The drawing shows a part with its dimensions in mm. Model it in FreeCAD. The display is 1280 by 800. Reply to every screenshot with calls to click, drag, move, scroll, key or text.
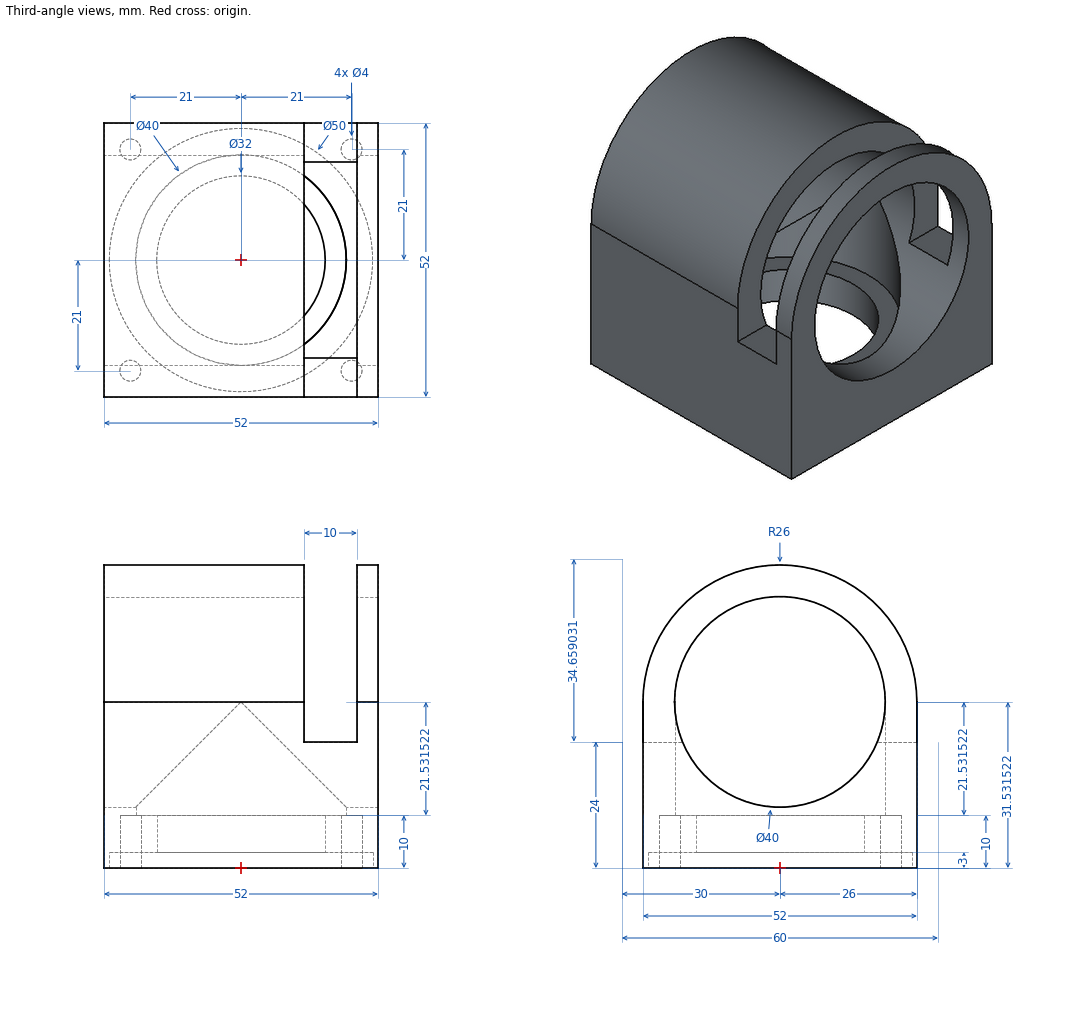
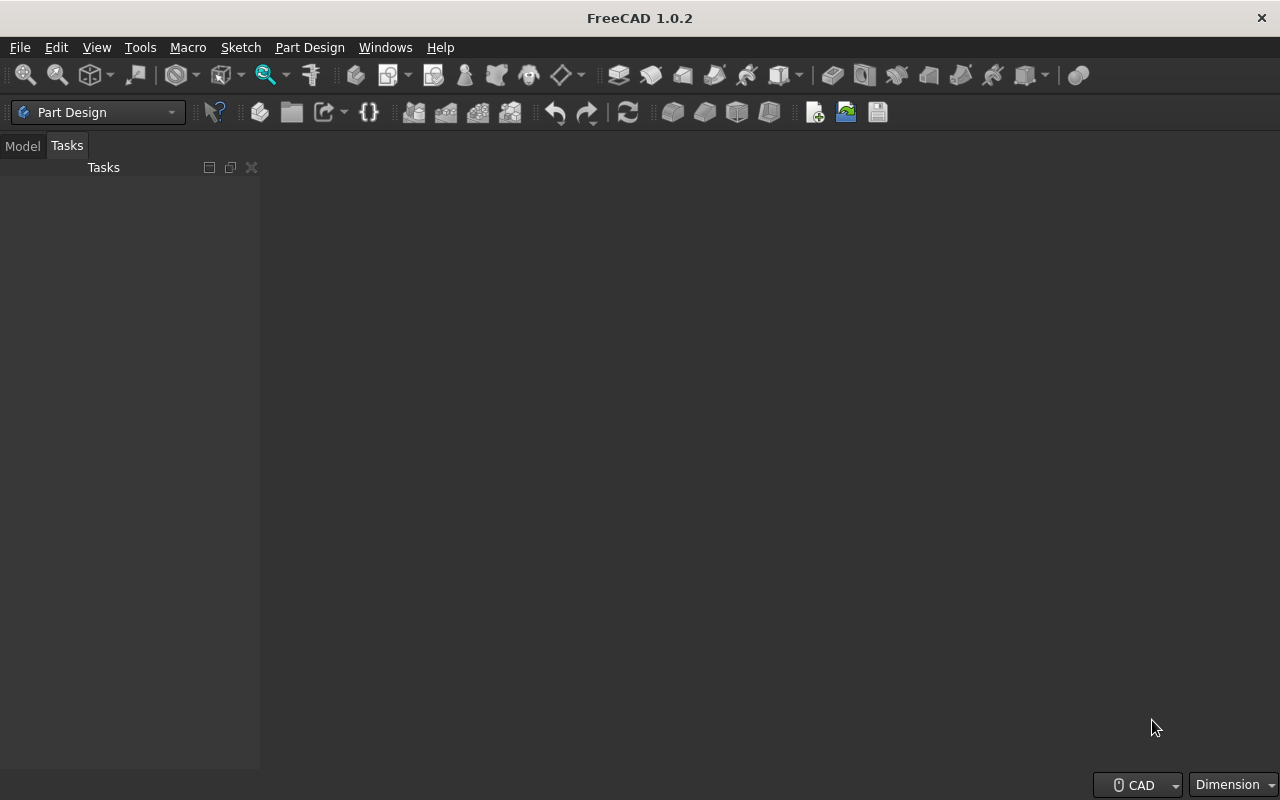
click(814, 112)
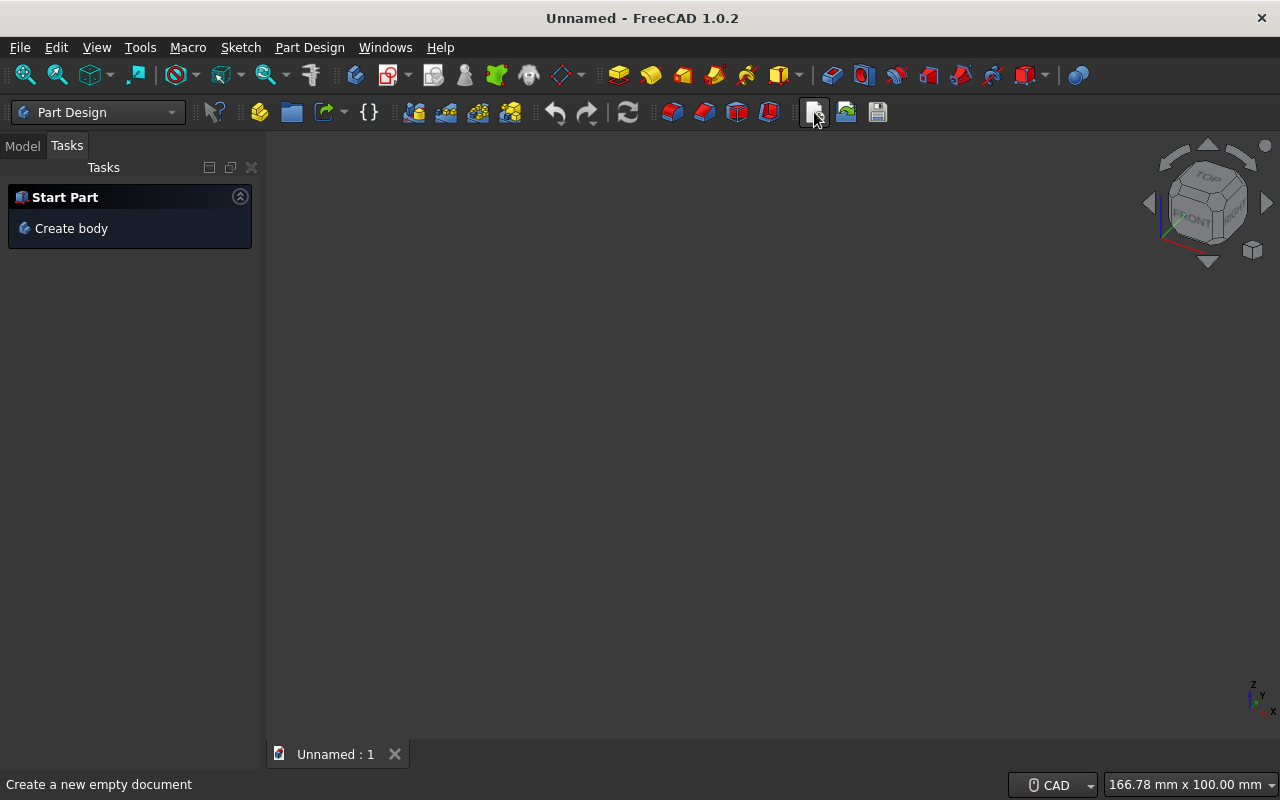
click(388, 76)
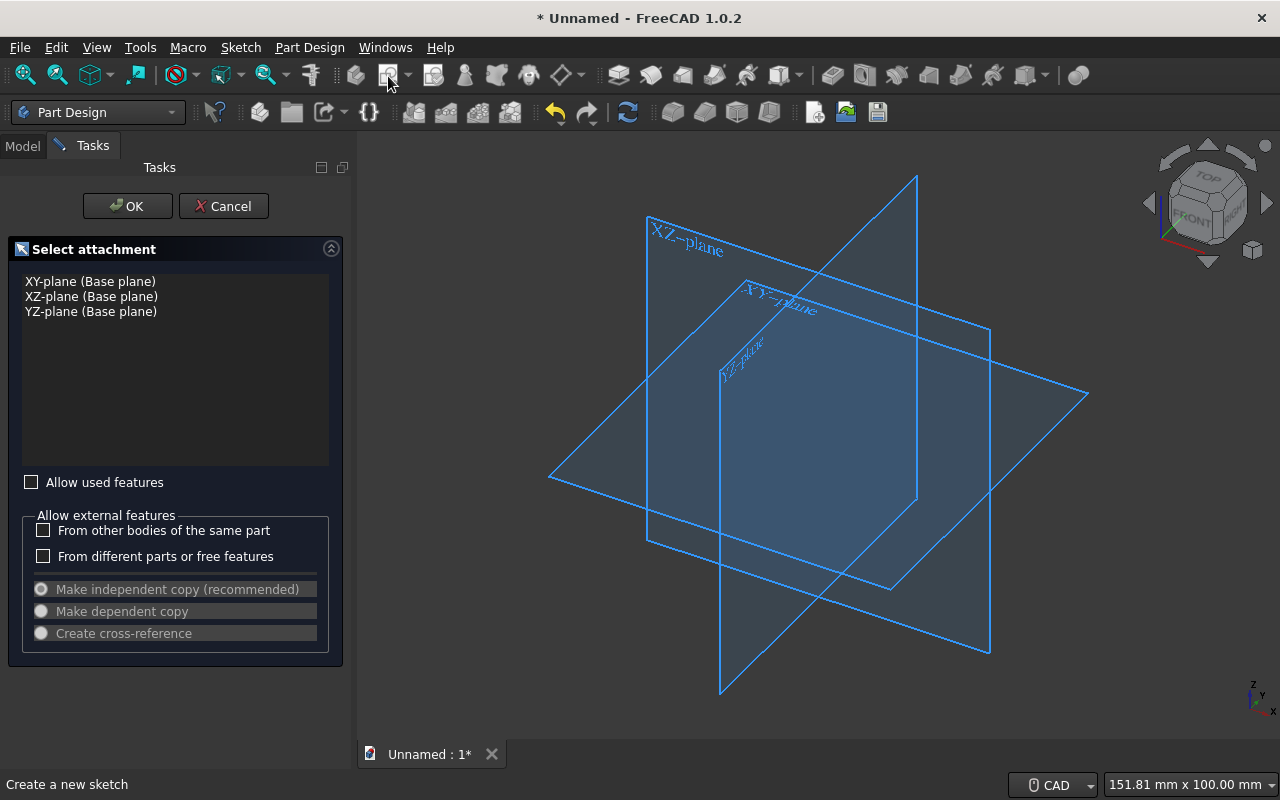
click(82, 282)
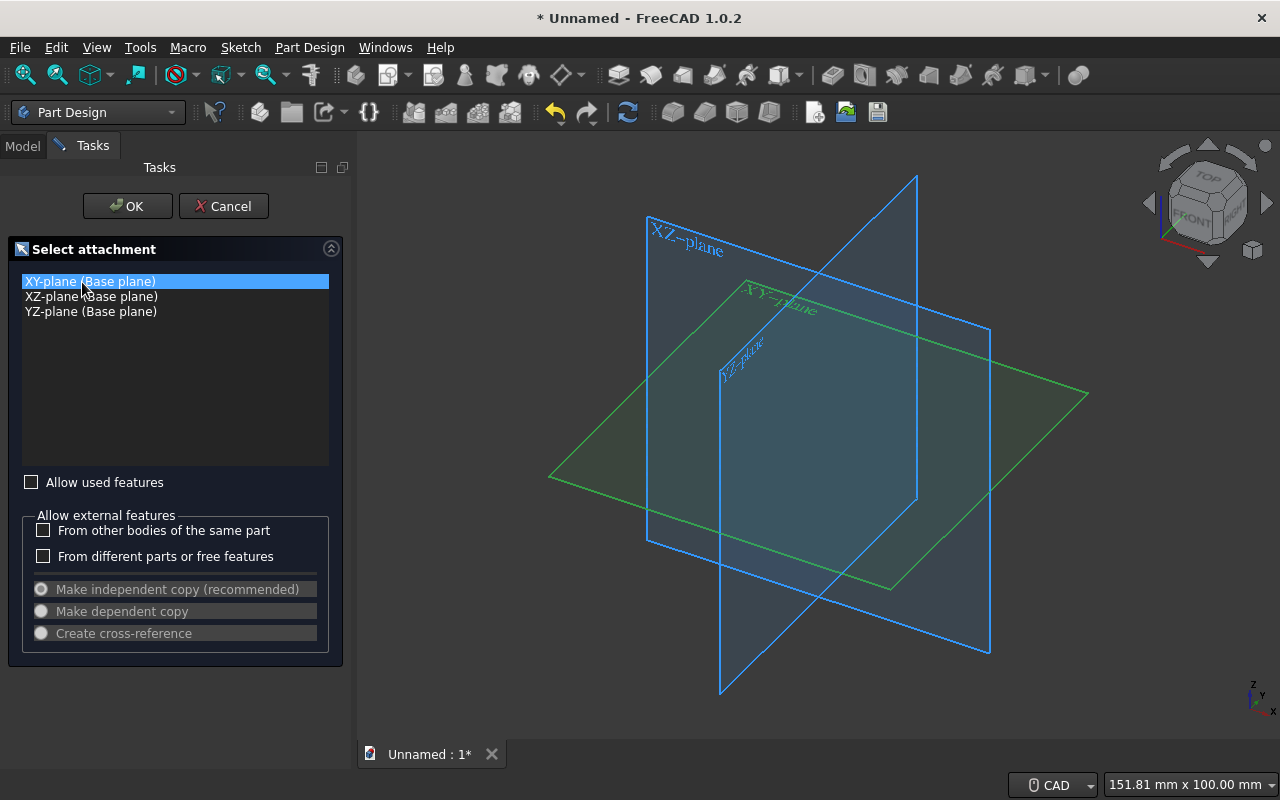
click(128, 206)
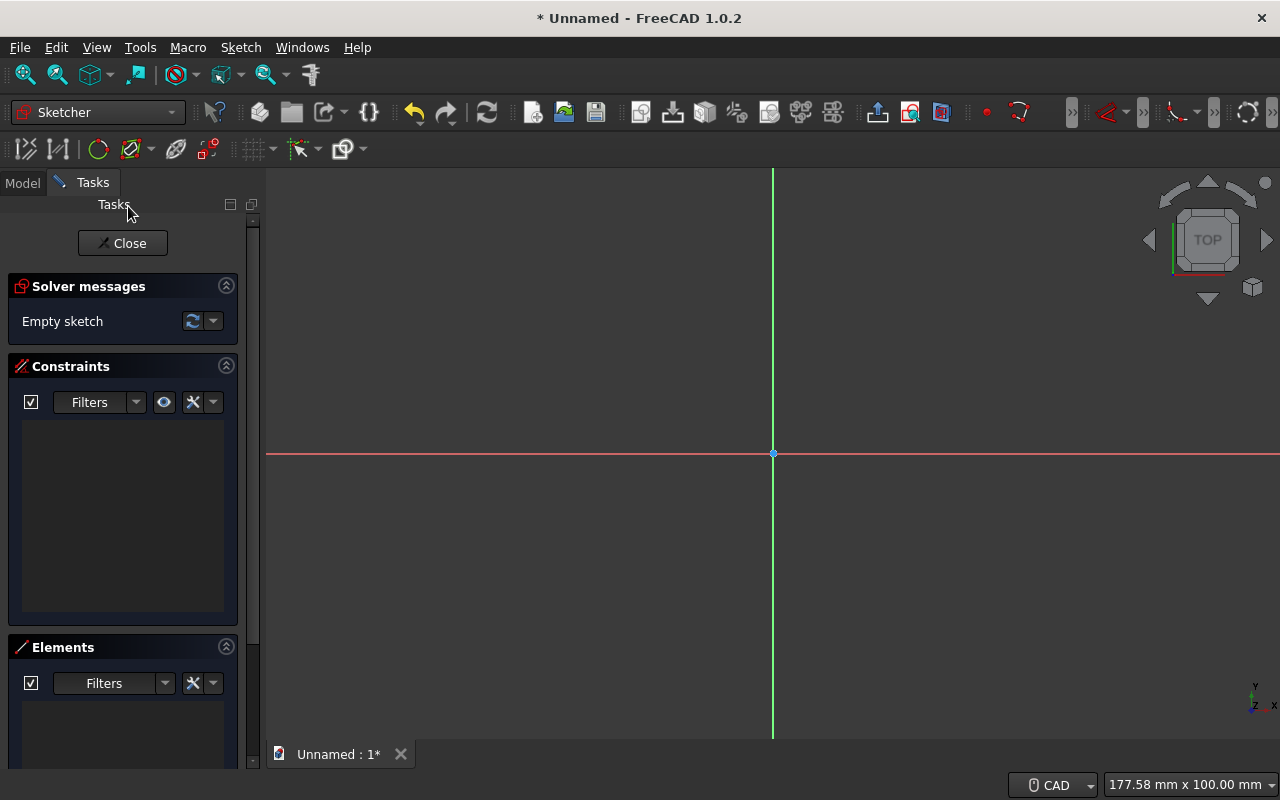
key(g)
key(v)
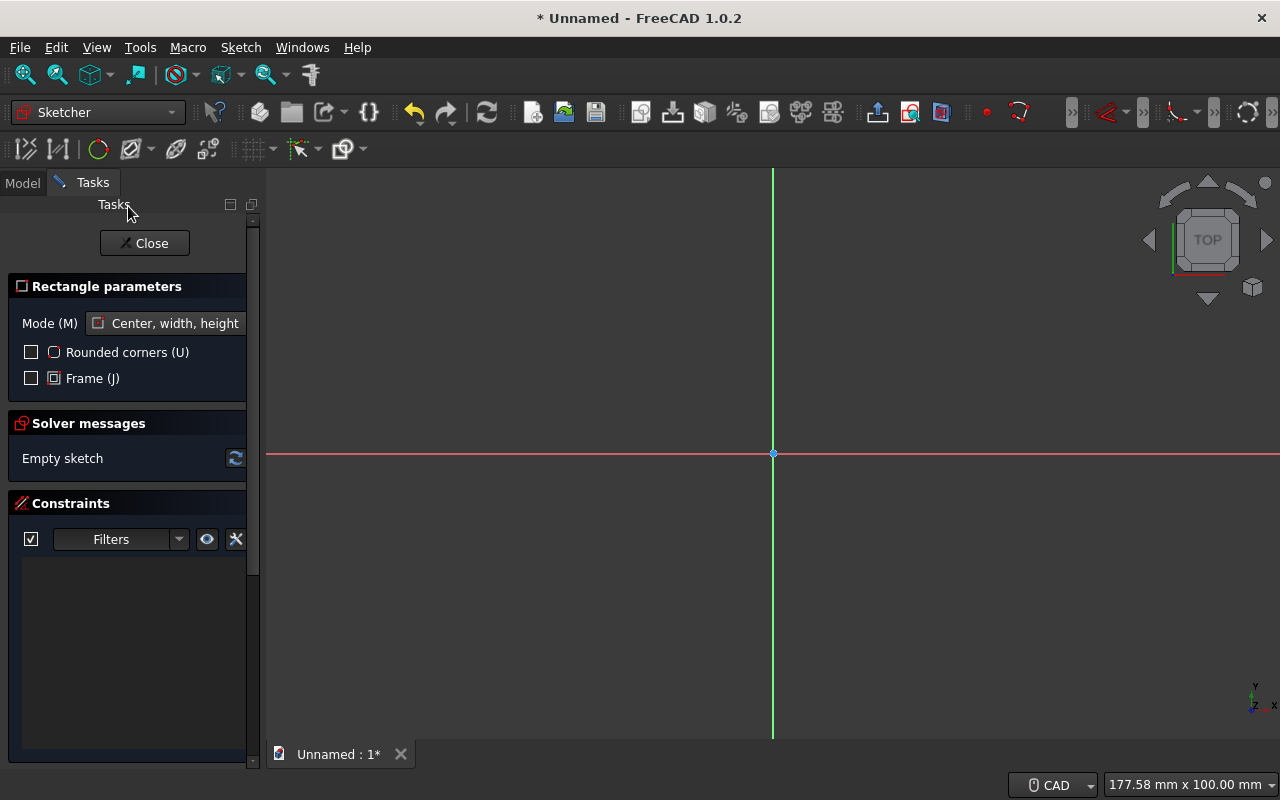
click(773, 454)
click(921, 305)
key(Escape)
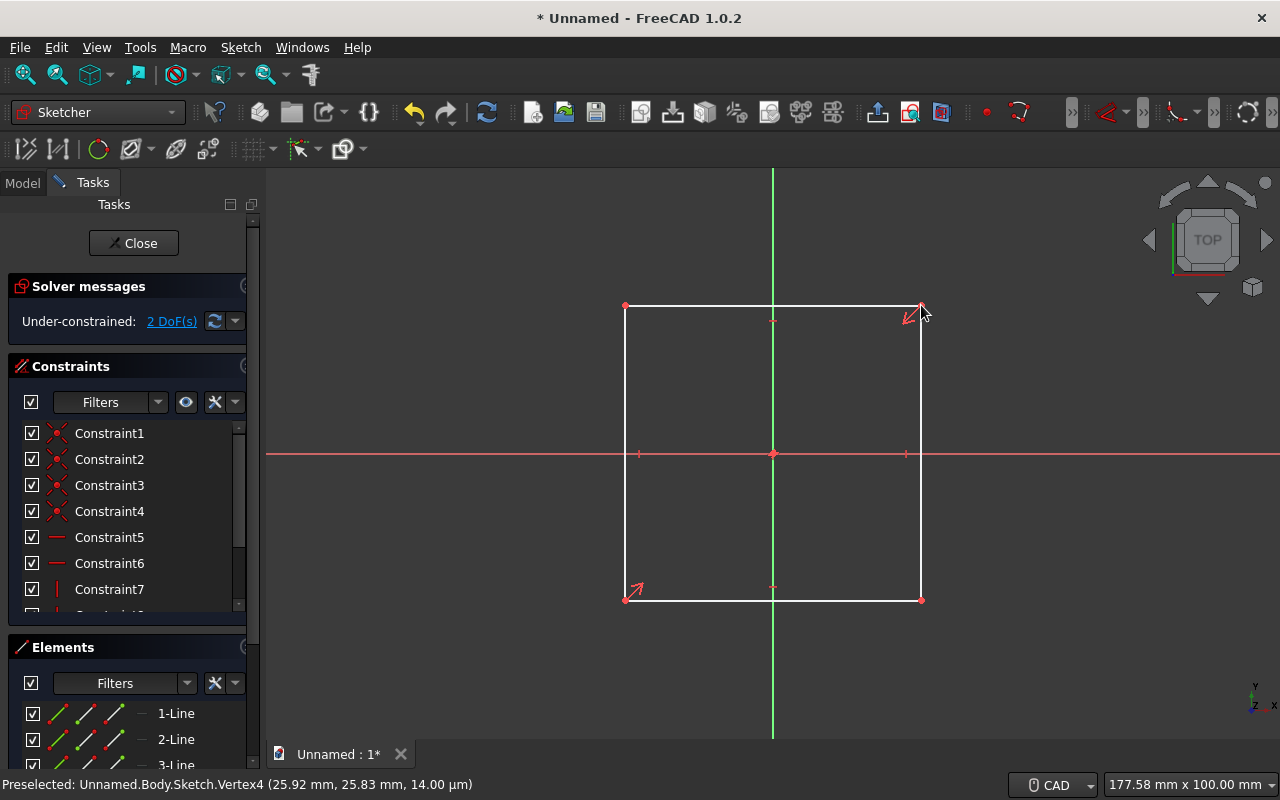
click(1106, 112)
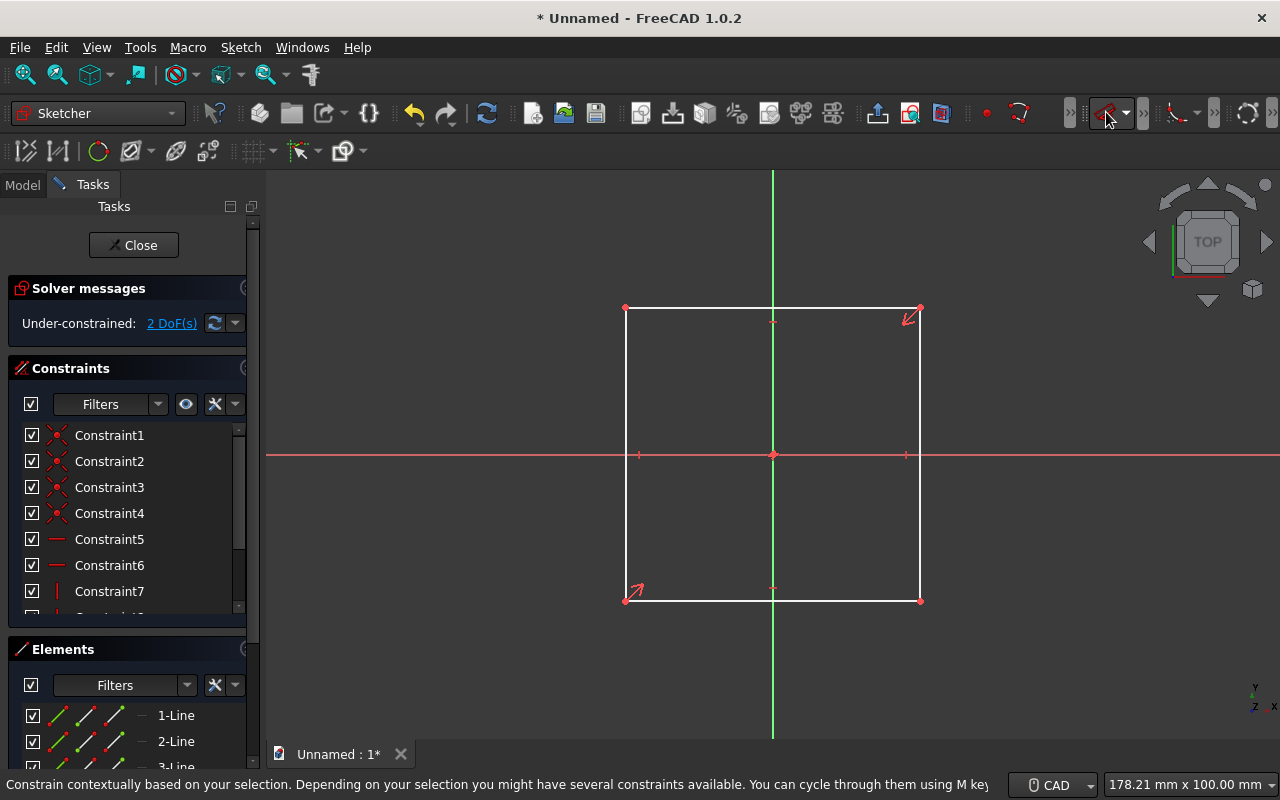
click(714, 601)
click(705, 635)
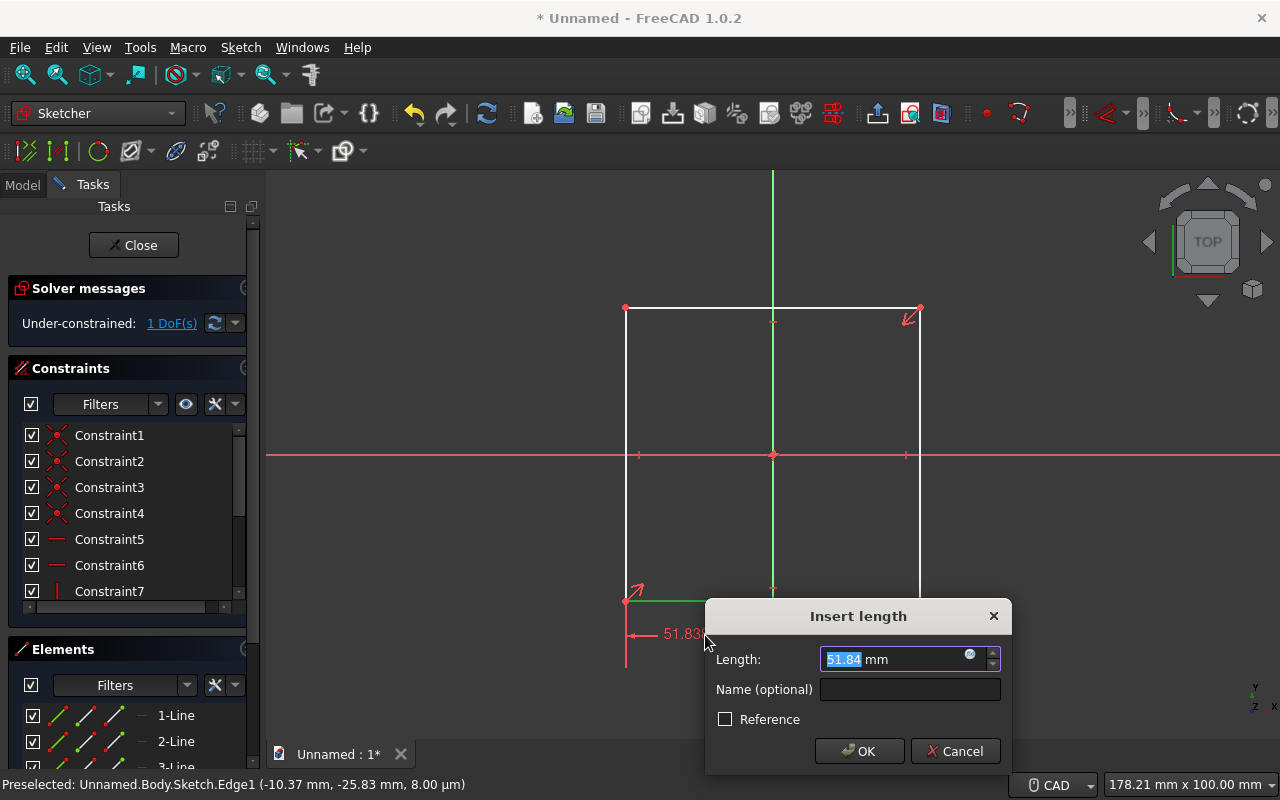
text(52)
key(Return)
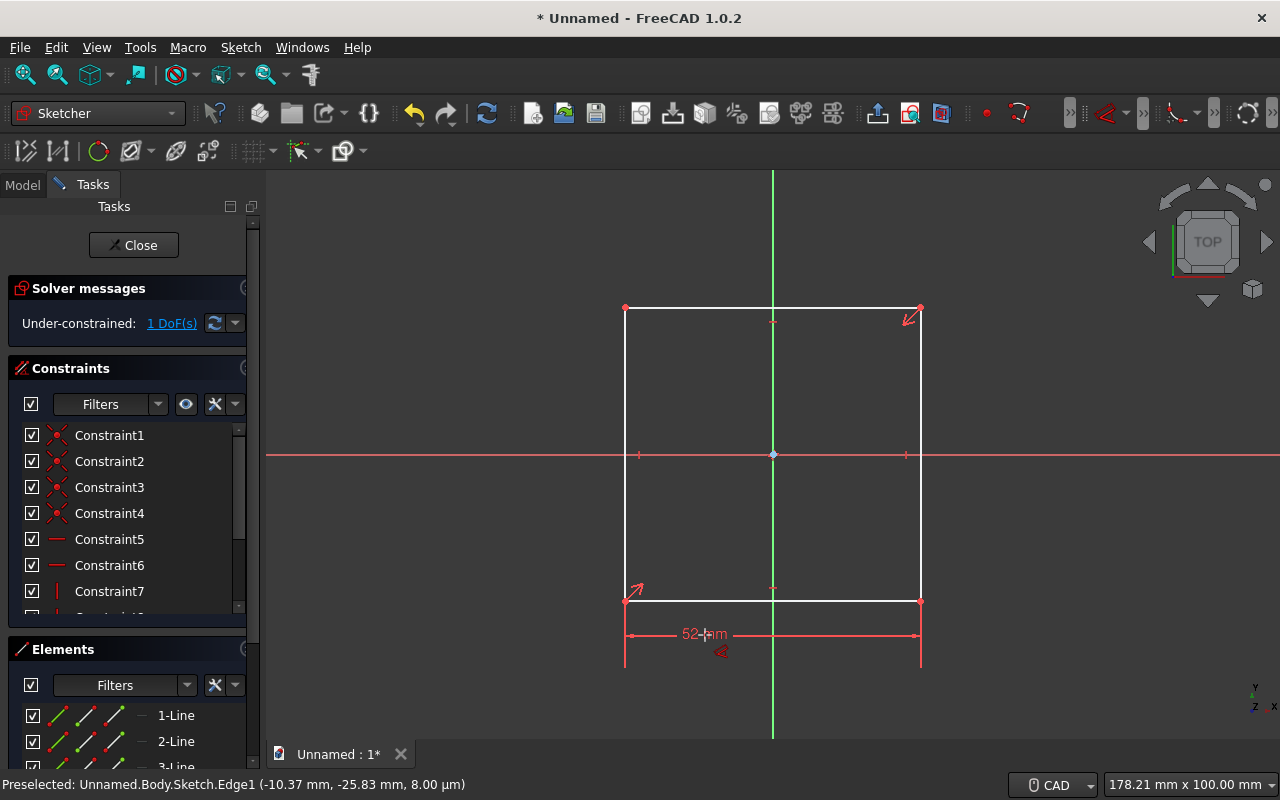
click(921, 513)
click(955, 387)